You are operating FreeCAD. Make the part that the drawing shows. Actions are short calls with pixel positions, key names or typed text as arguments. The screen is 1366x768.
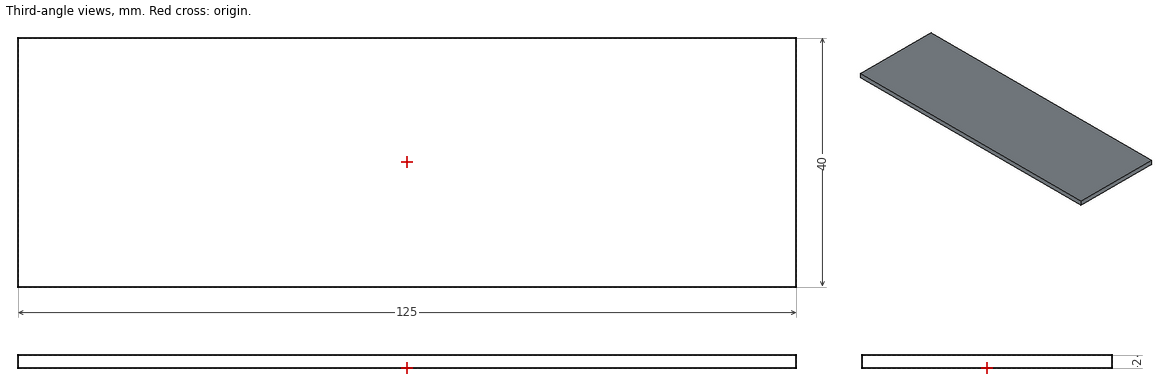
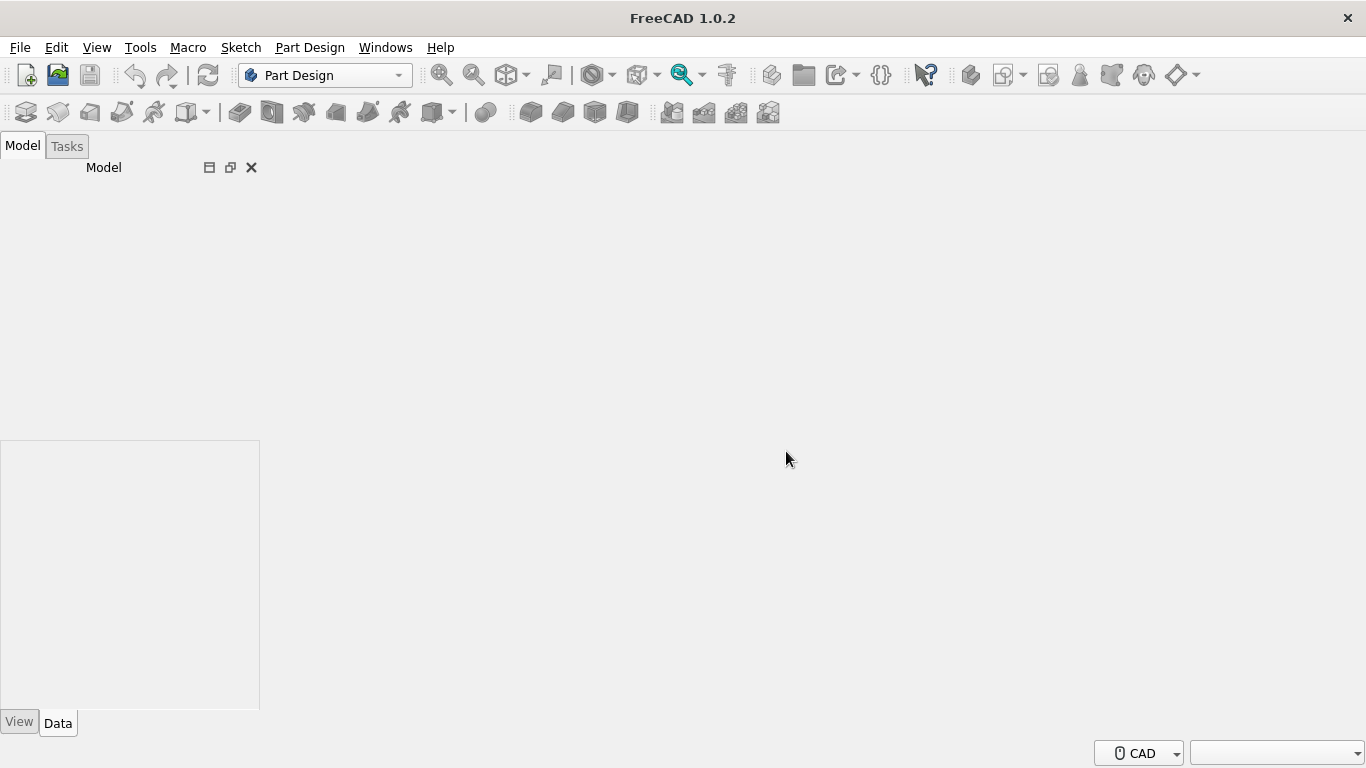
click(26, 76)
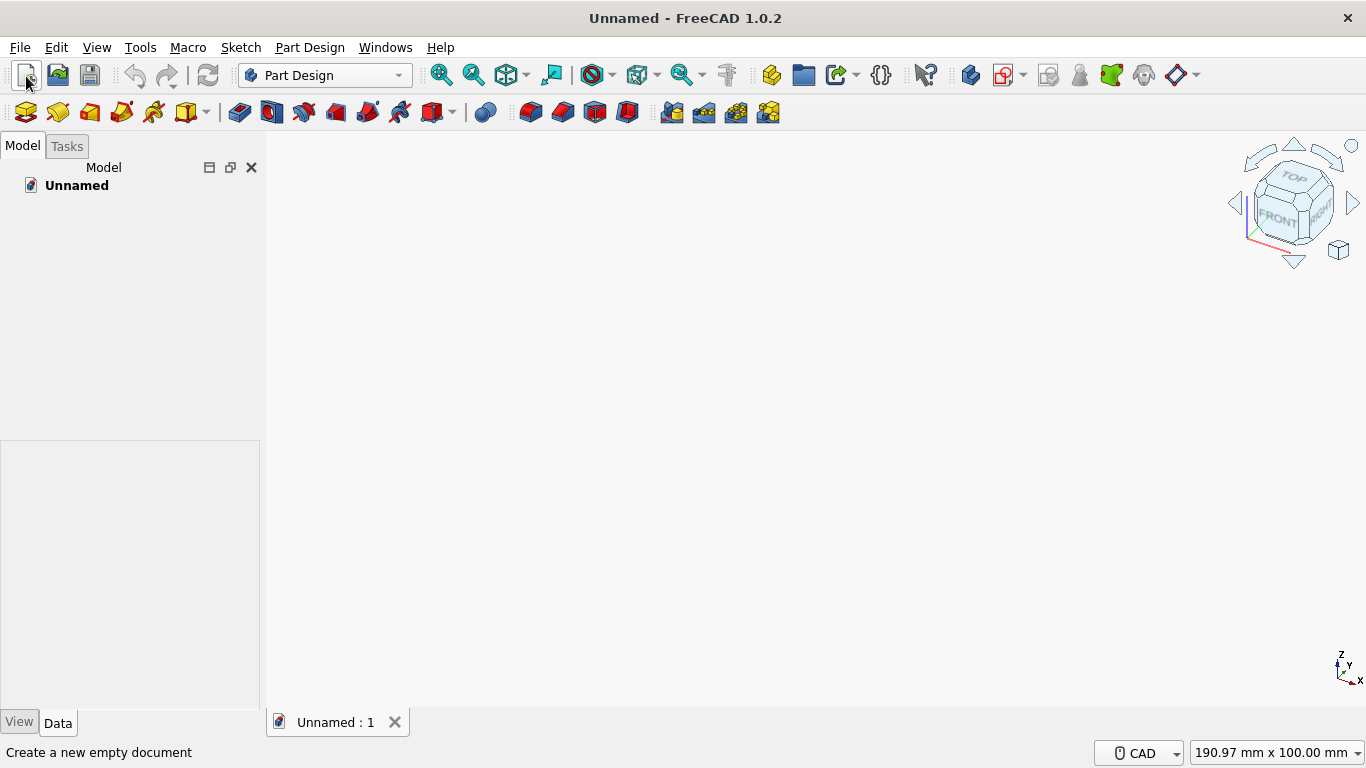
click(1004, 76)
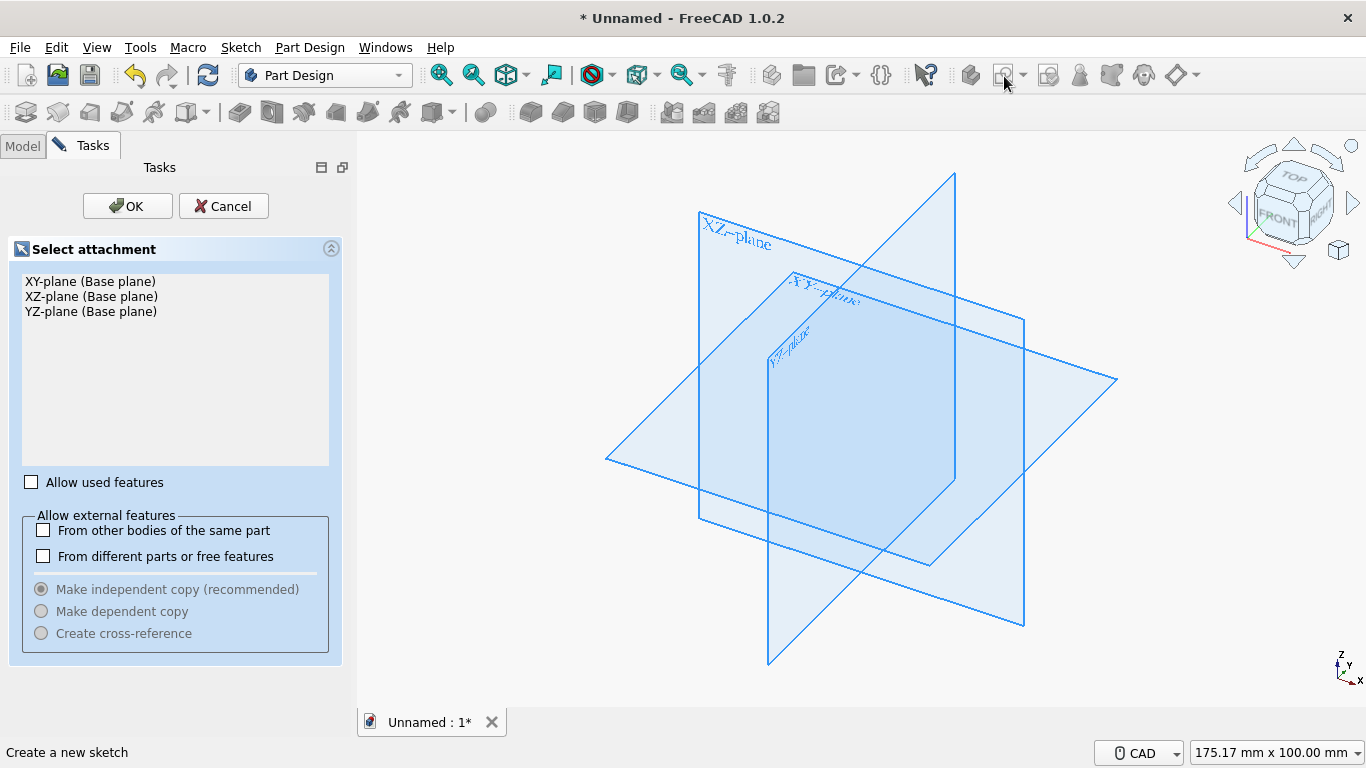
click(82, 282)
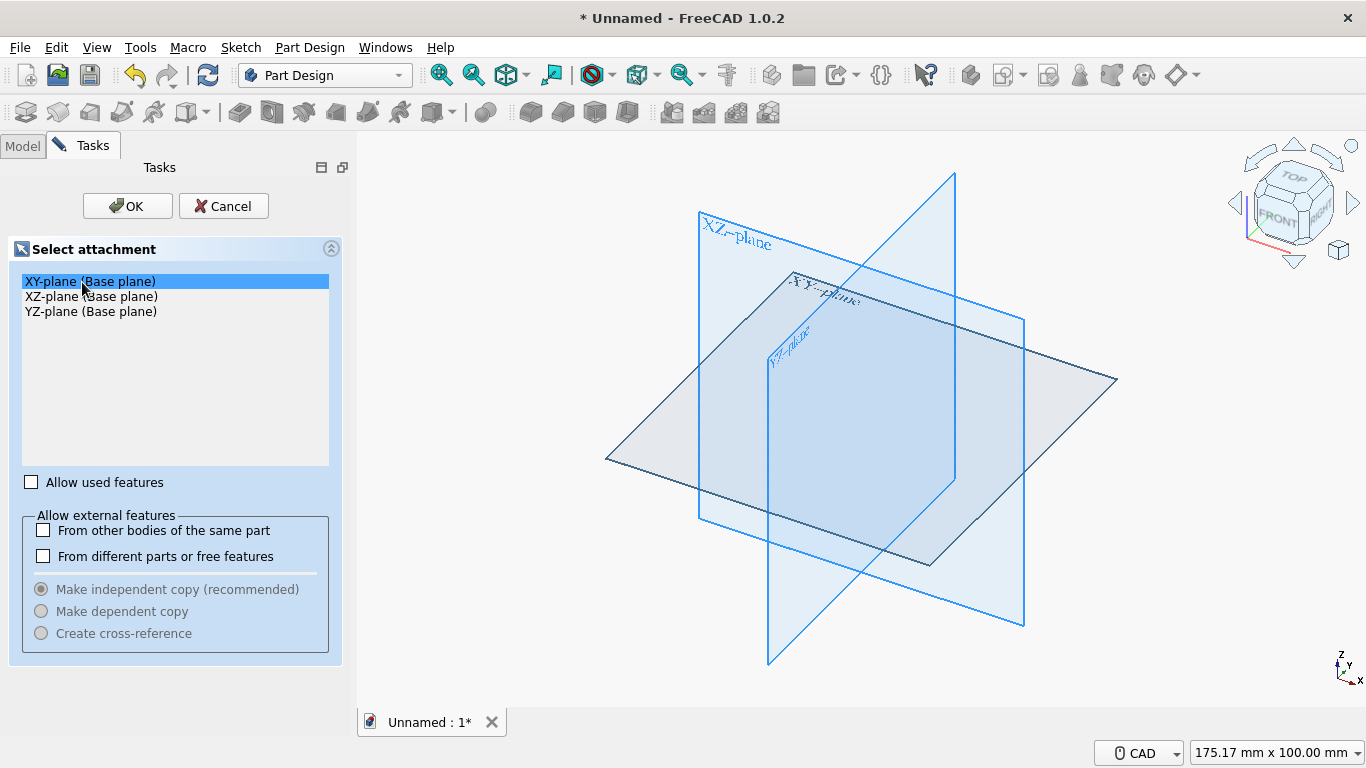
click(128, 206)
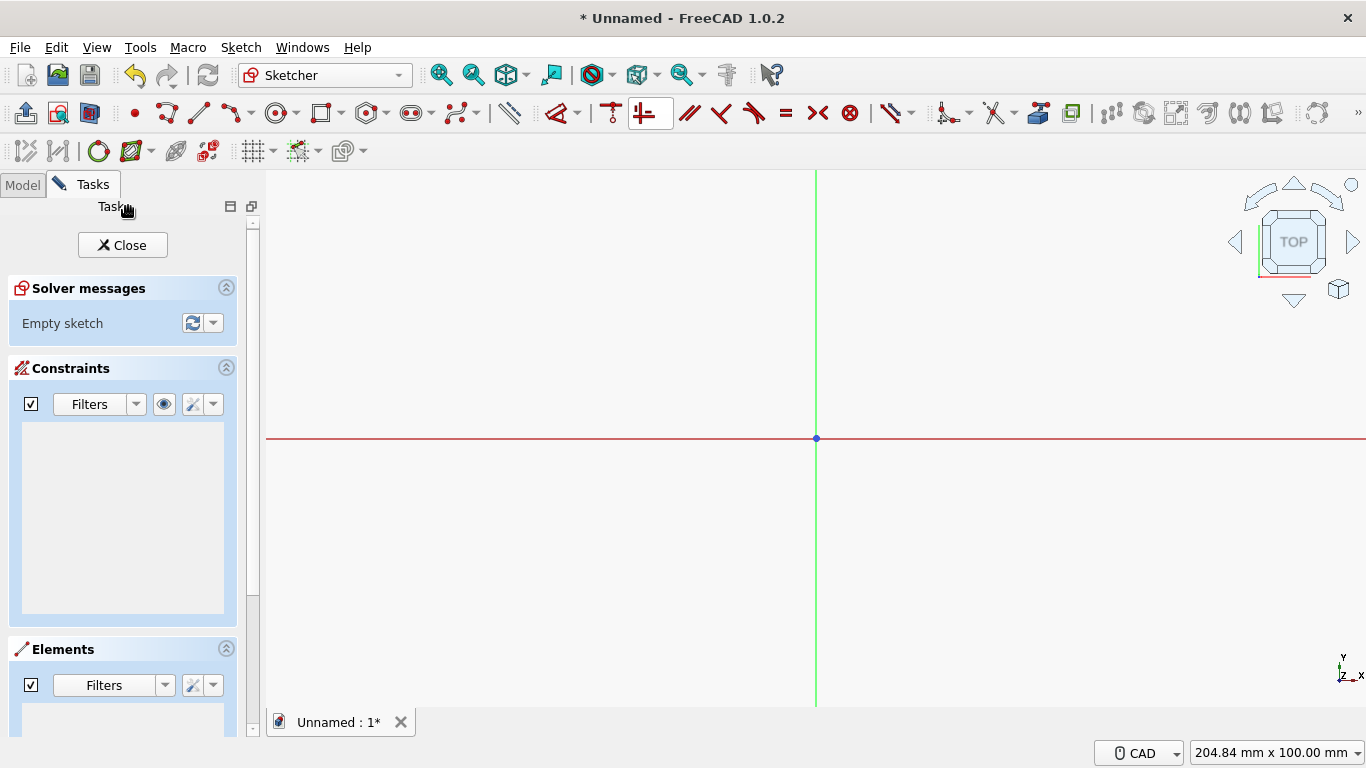
key(g)
key(v)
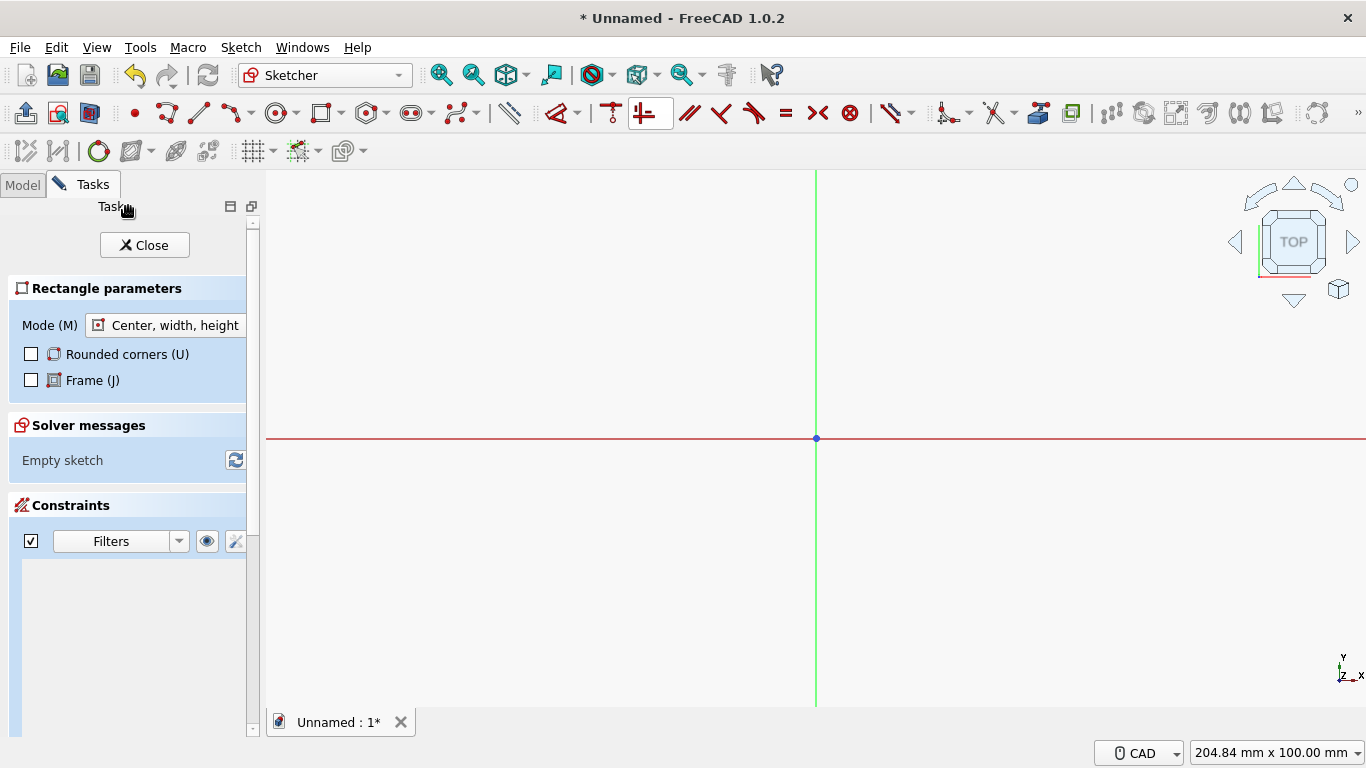
click(816, 438)
click(1152, 331)
key(Escape)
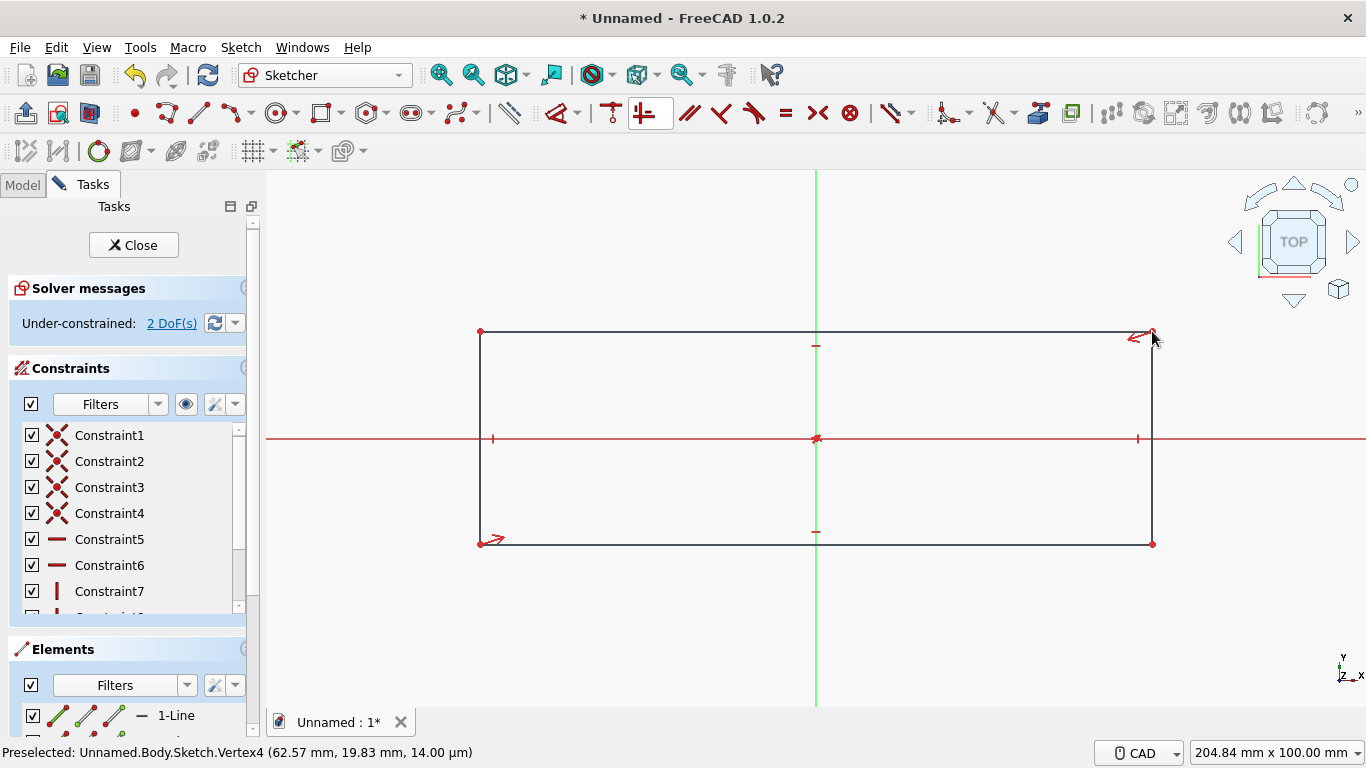
key(d)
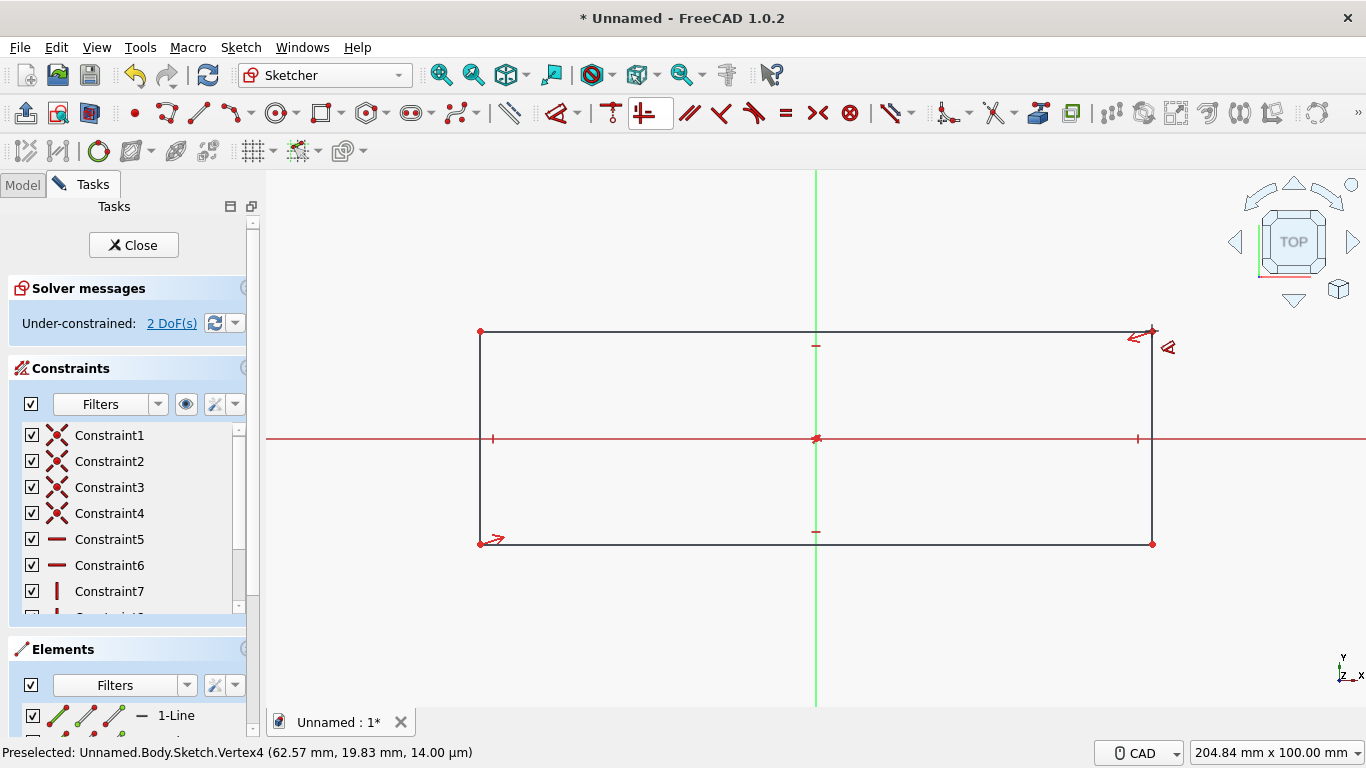
click(1152, 481)
click(1186, 390)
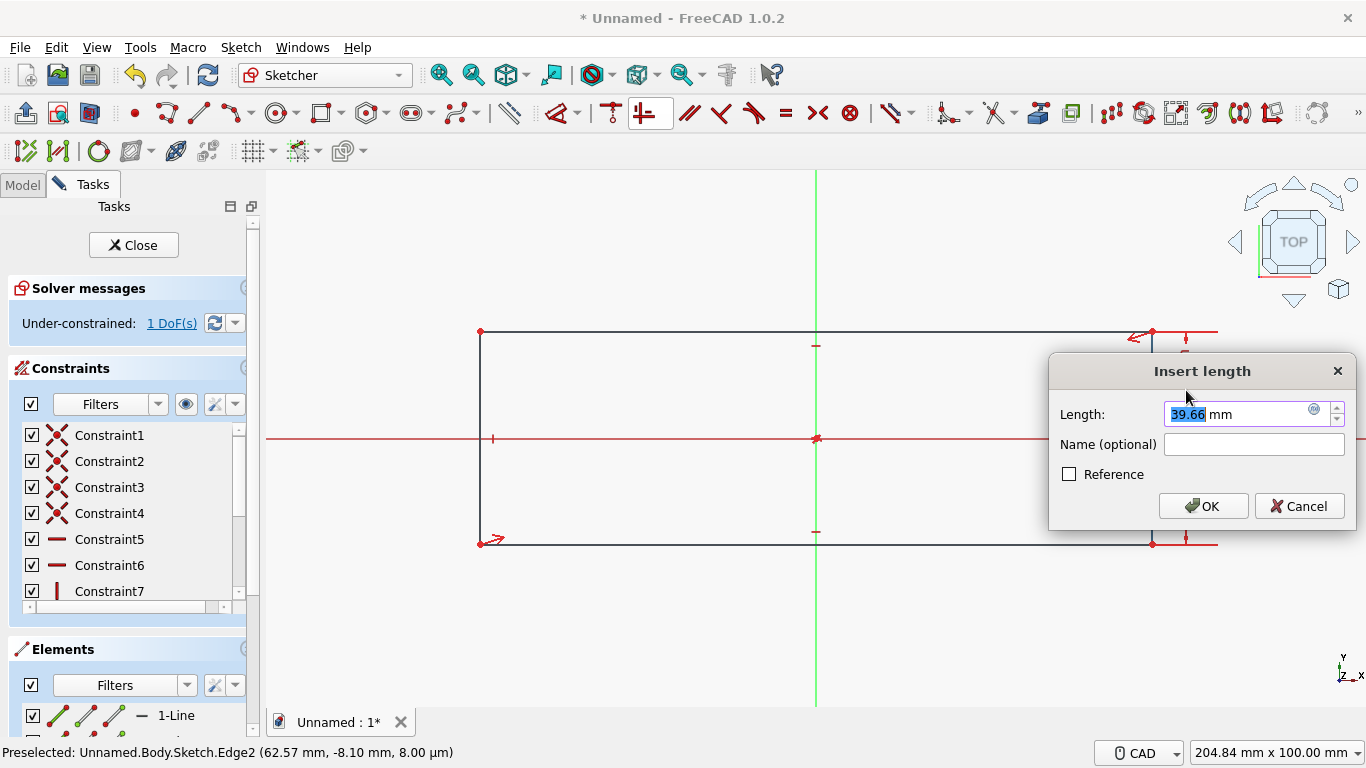
text(40)
key(Return)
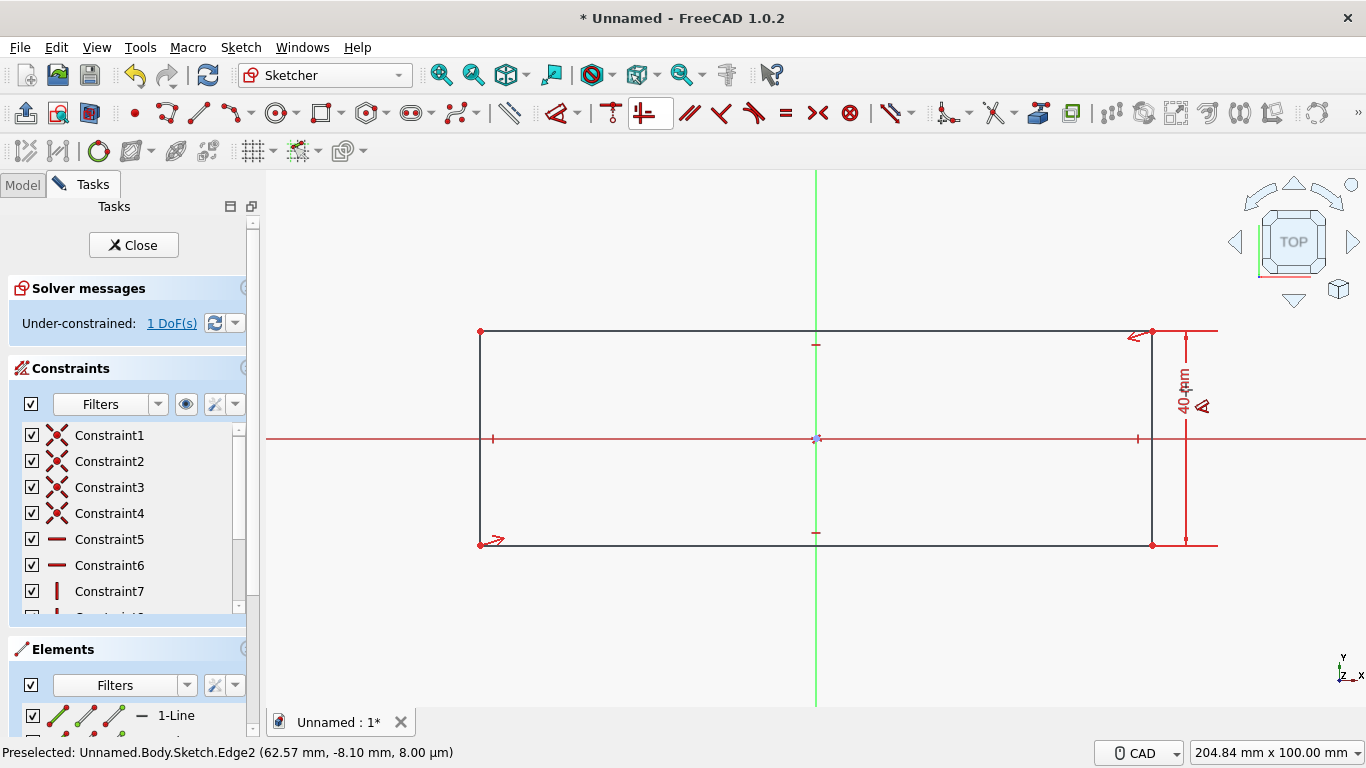
click(682, 546)
click(661, 580)